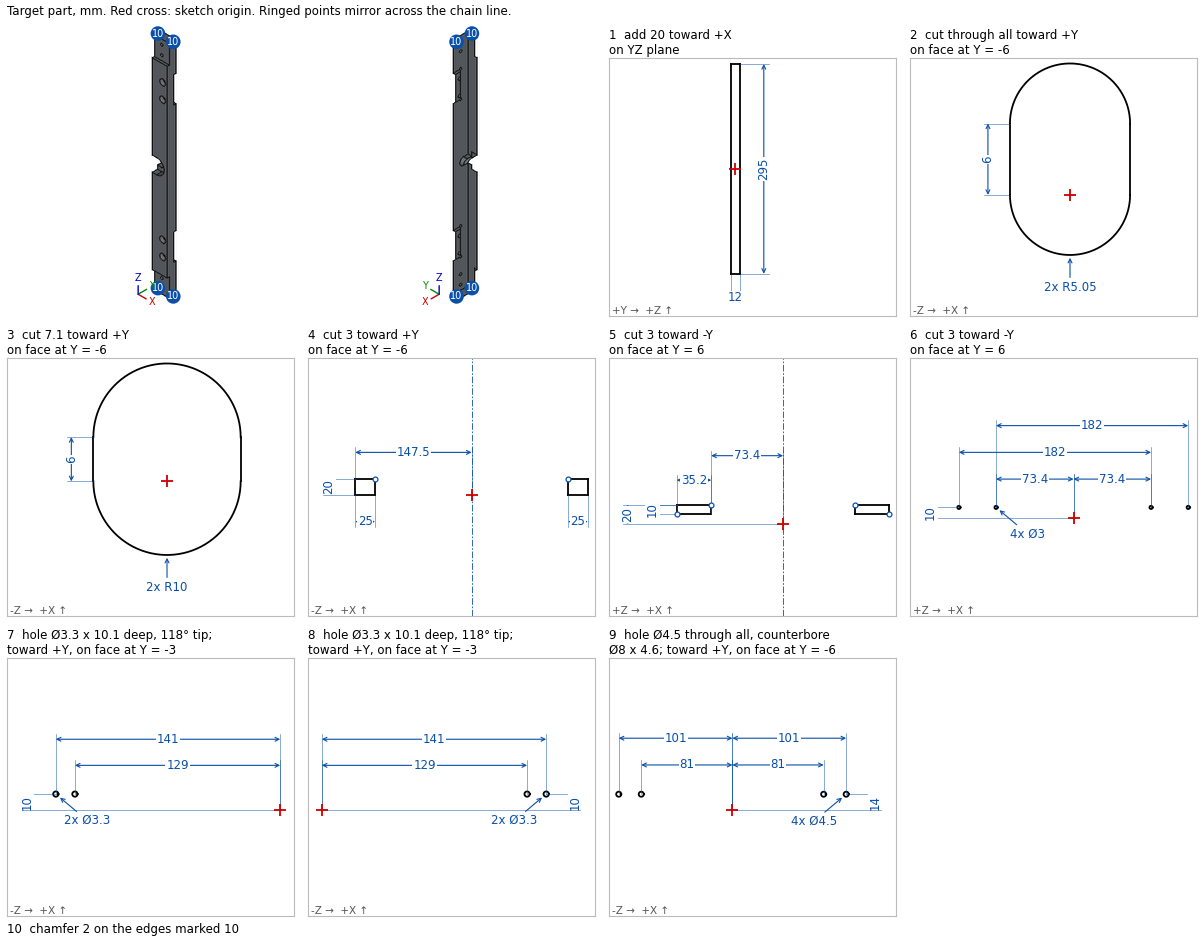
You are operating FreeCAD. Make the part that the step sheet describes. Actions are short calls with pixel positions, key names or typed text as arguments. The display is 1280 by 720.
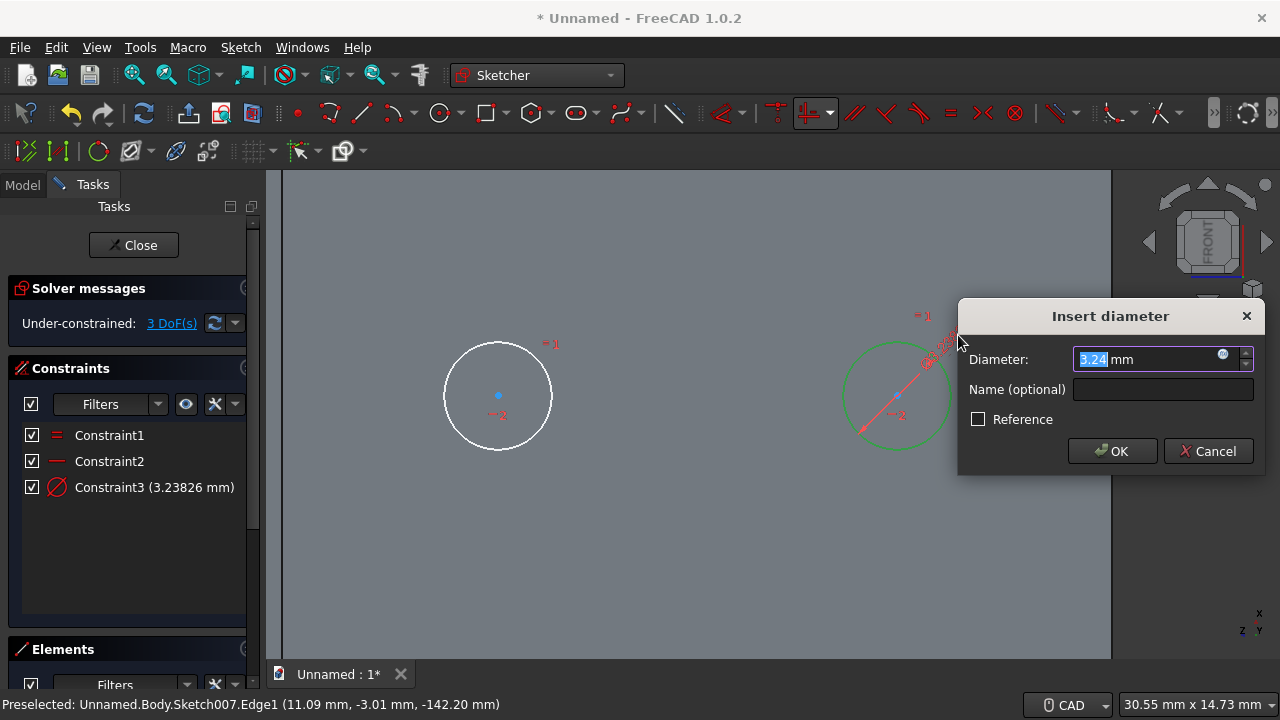
text(3.3)
key(Return)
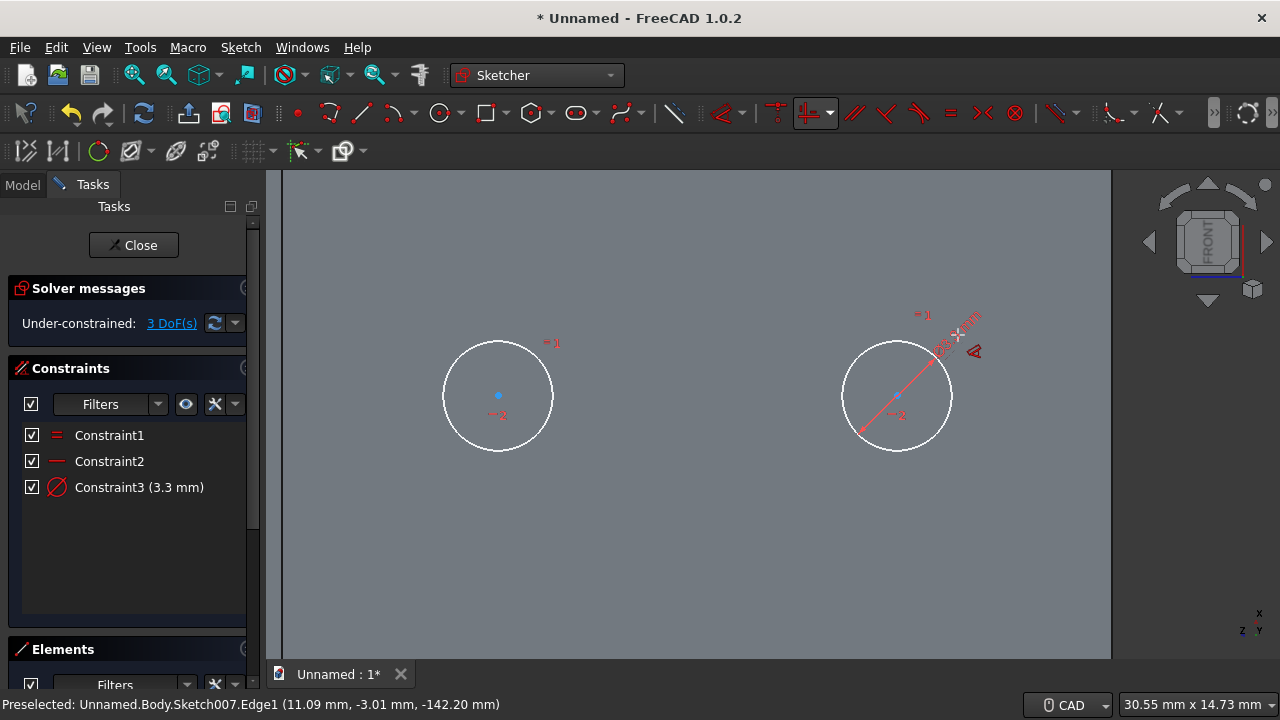
click(897, 396)
click(931, 513)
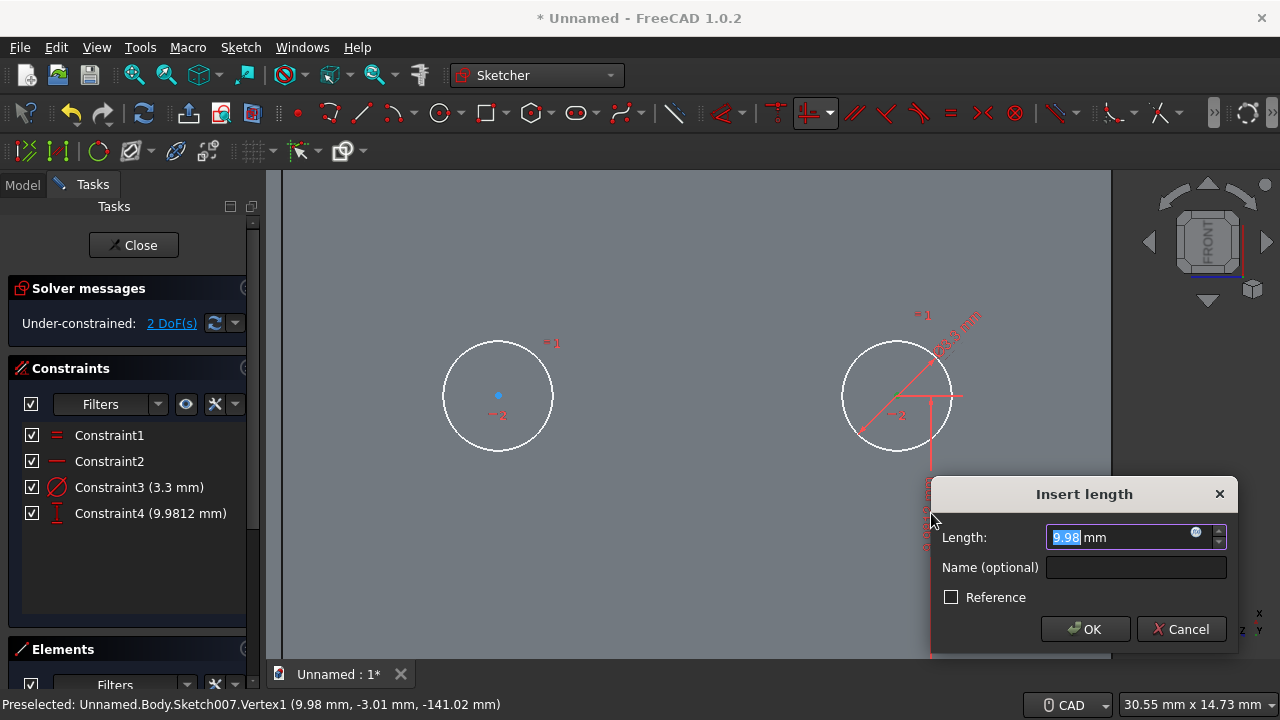
text(10)
key(Return)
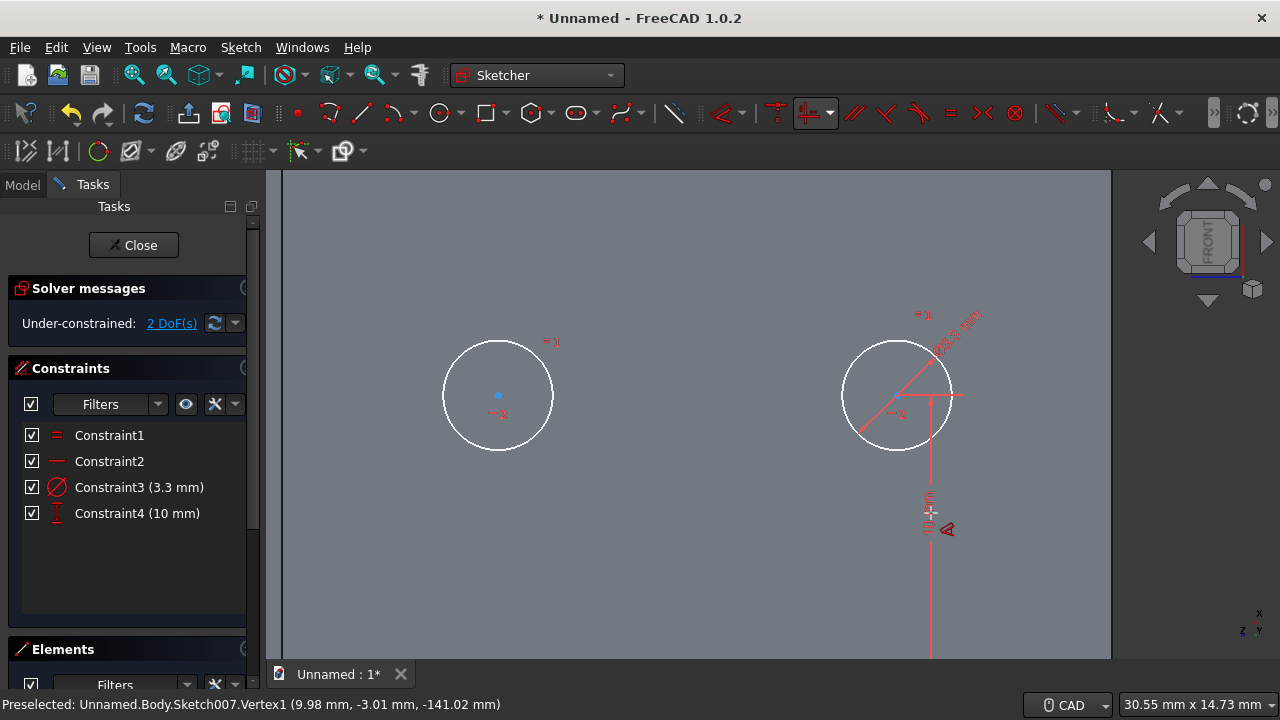
click(897, 395)
click(595, 361)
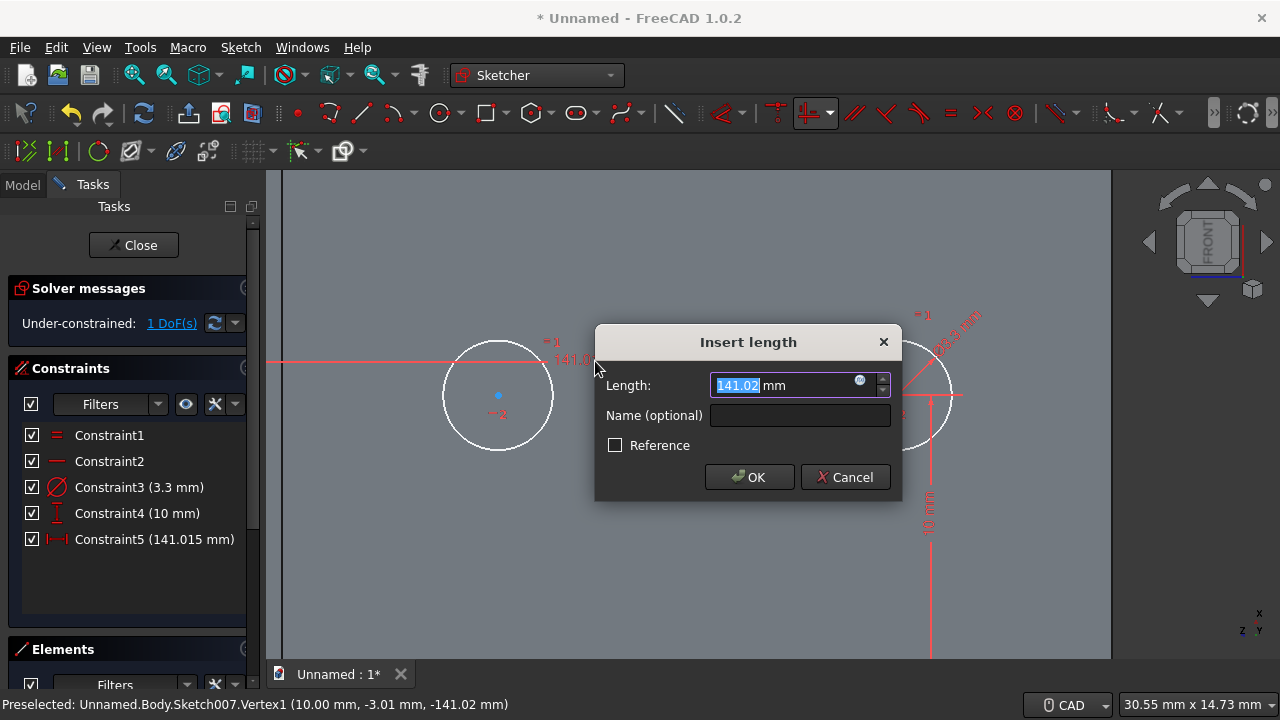
text(141)
key(Return)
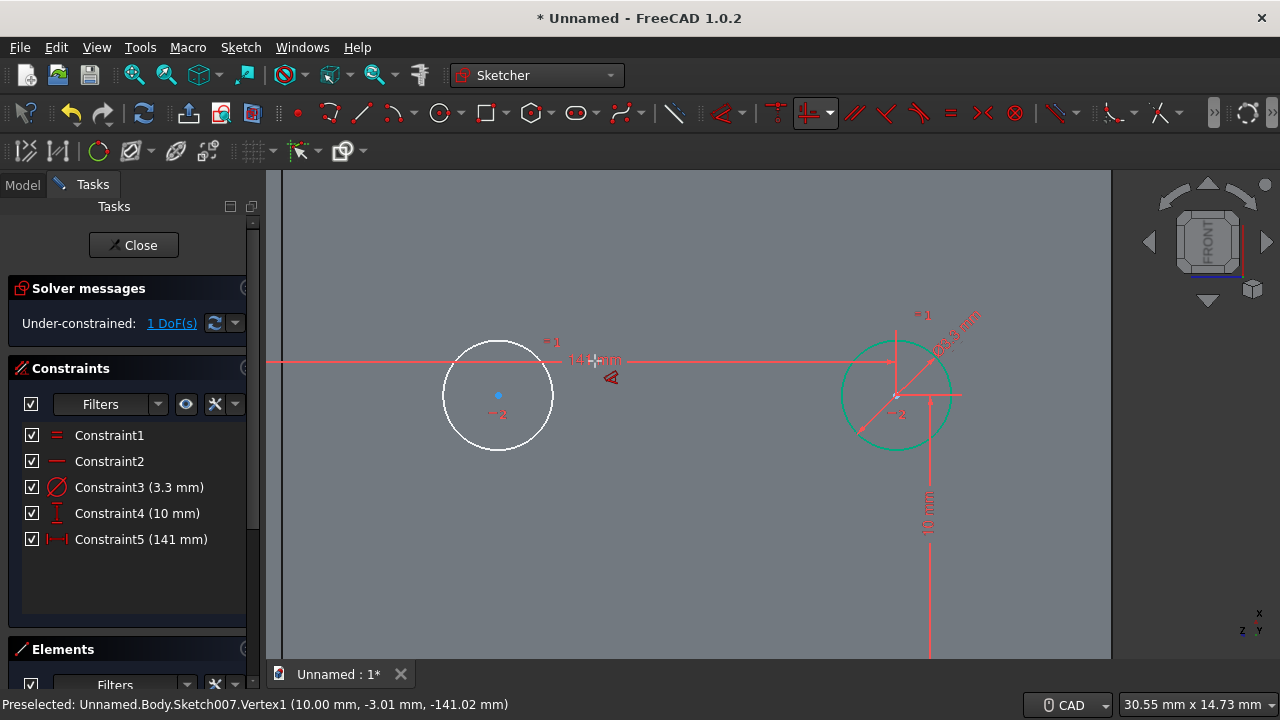
click(498, 395)
click(396, 361)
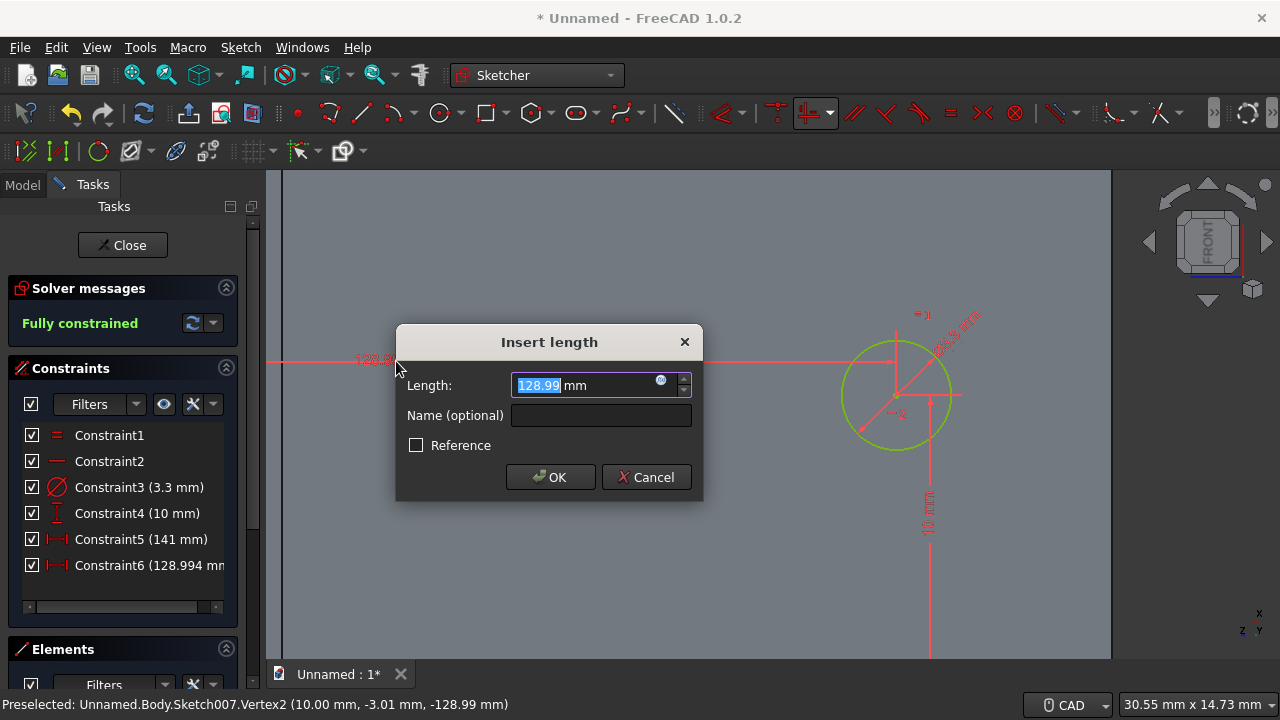
text(129)
key(Return)
key(Escape)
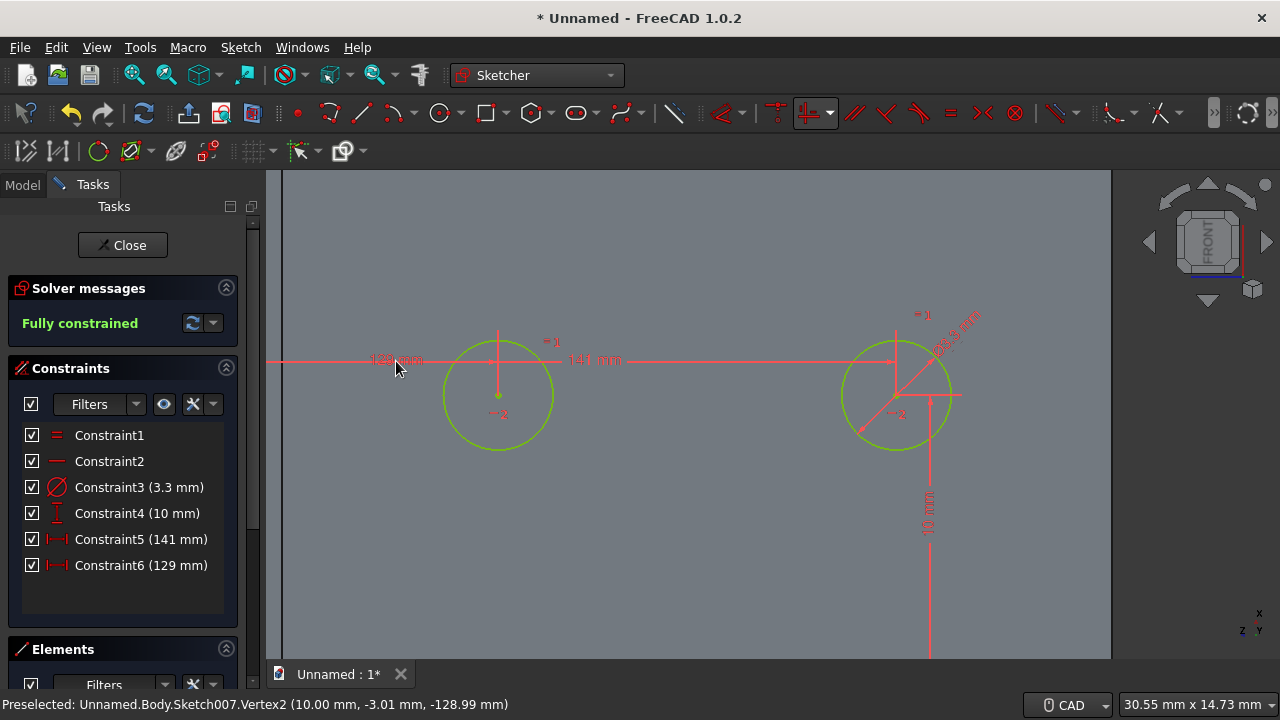
click(123, 245)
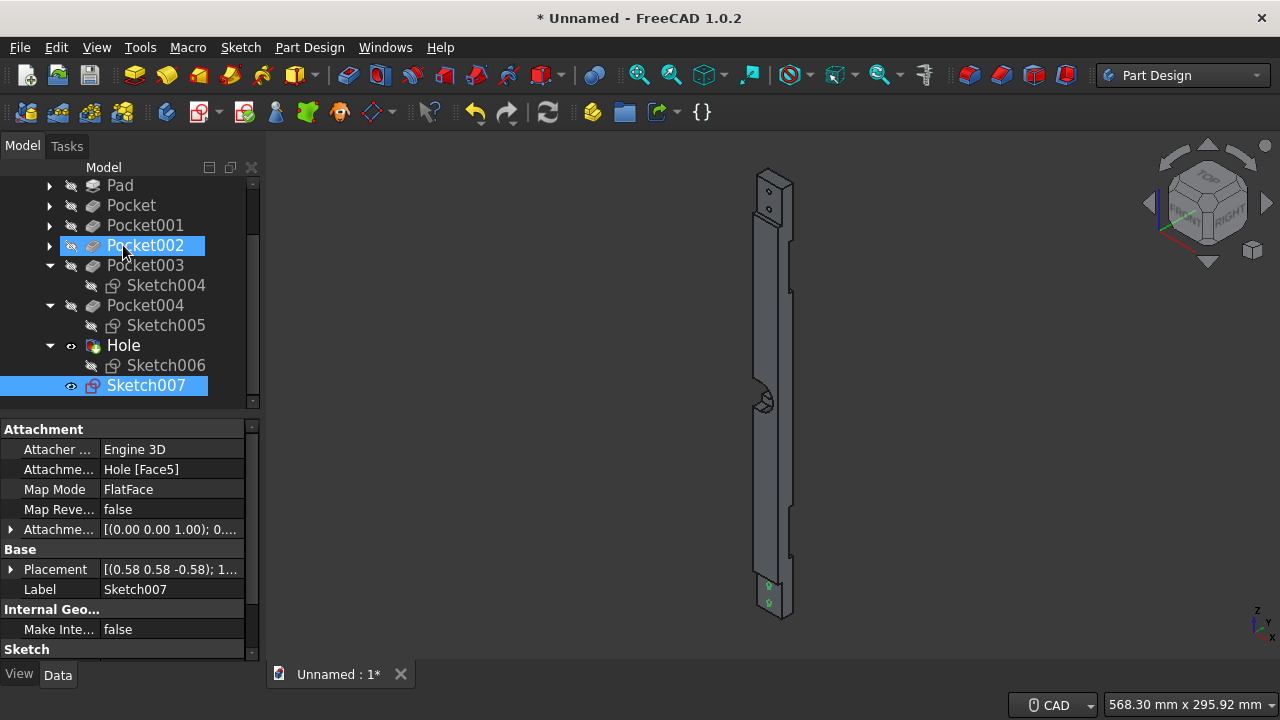
click(382, 76)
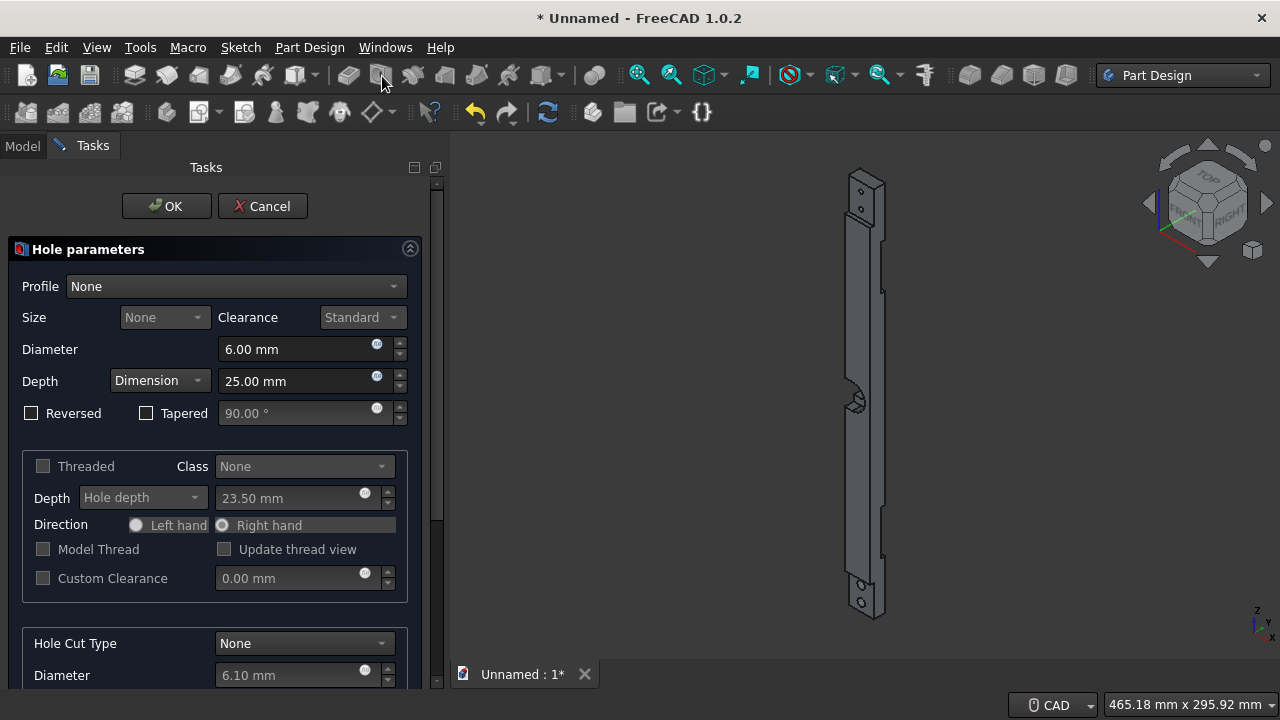
triple_click(305, 349)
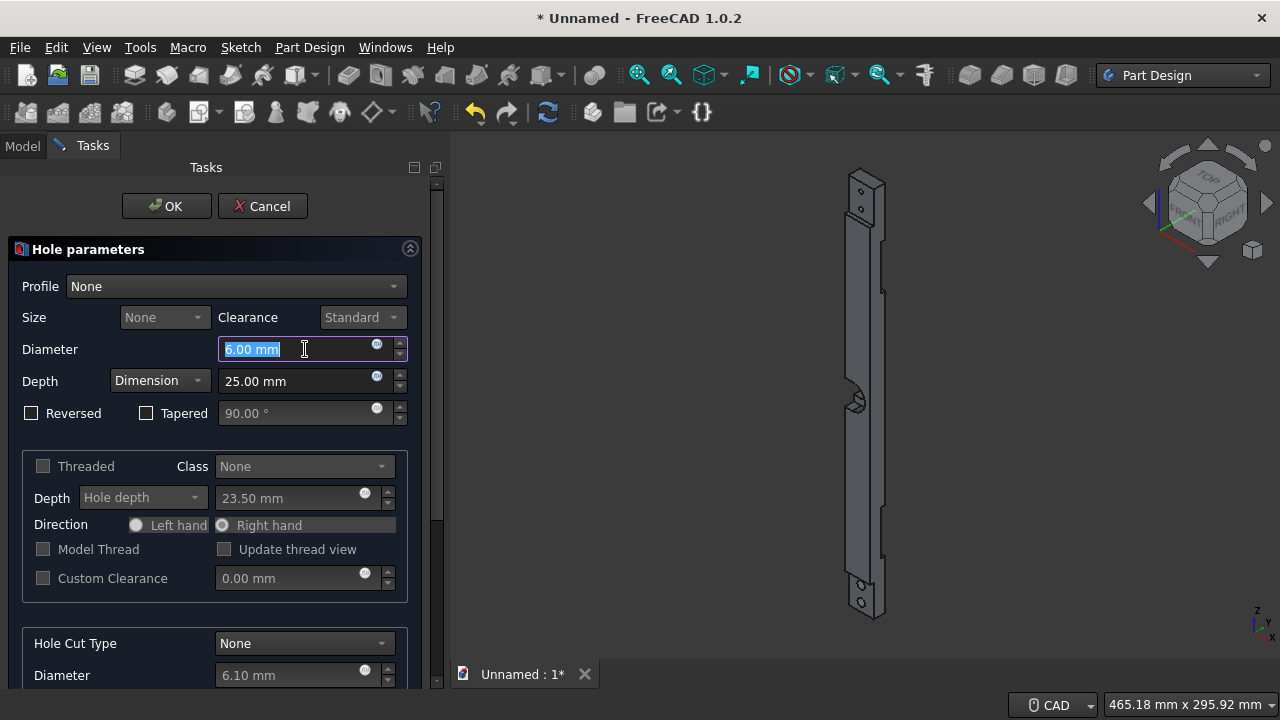
text(3.3)
key(Tab)